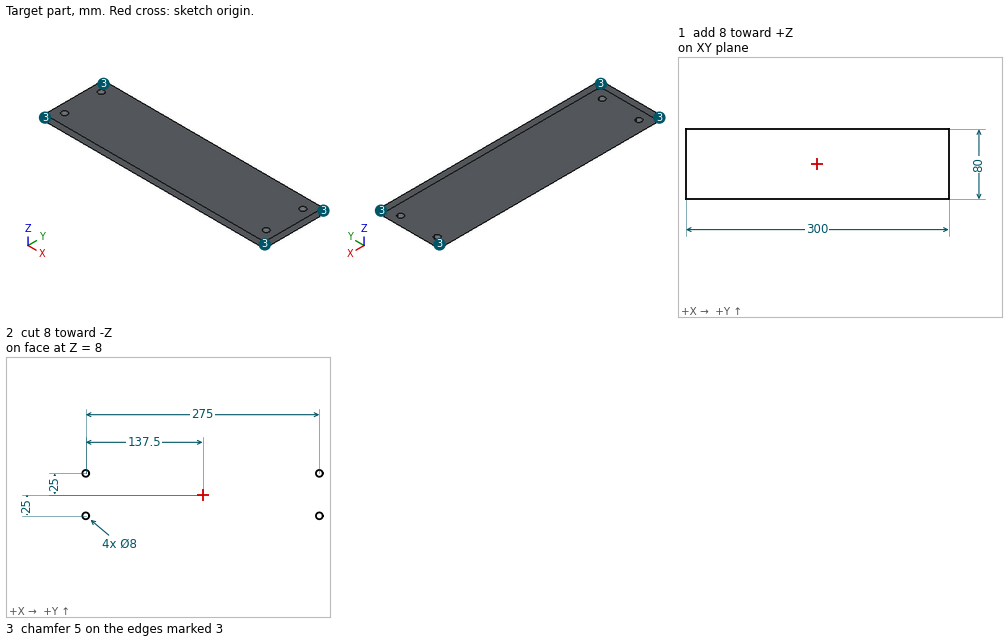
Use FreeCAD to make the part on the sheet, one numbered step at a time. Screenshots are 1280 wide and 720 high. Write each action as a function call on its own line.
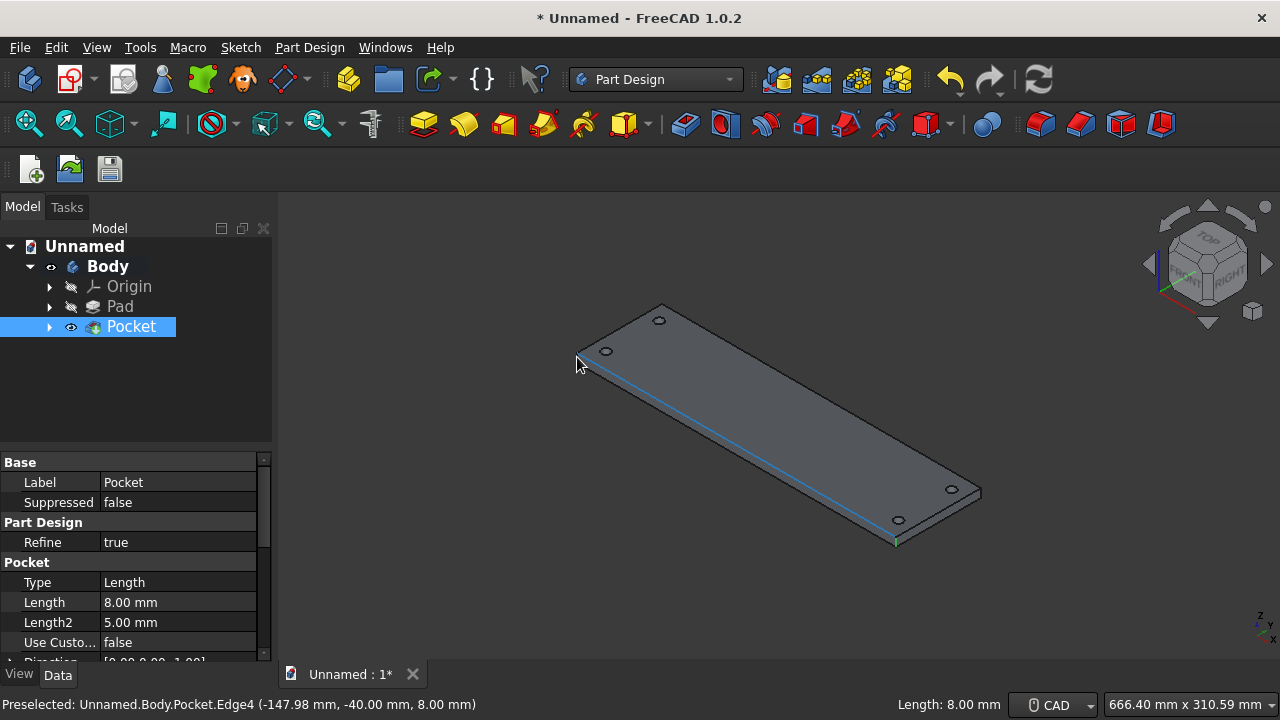
key(2)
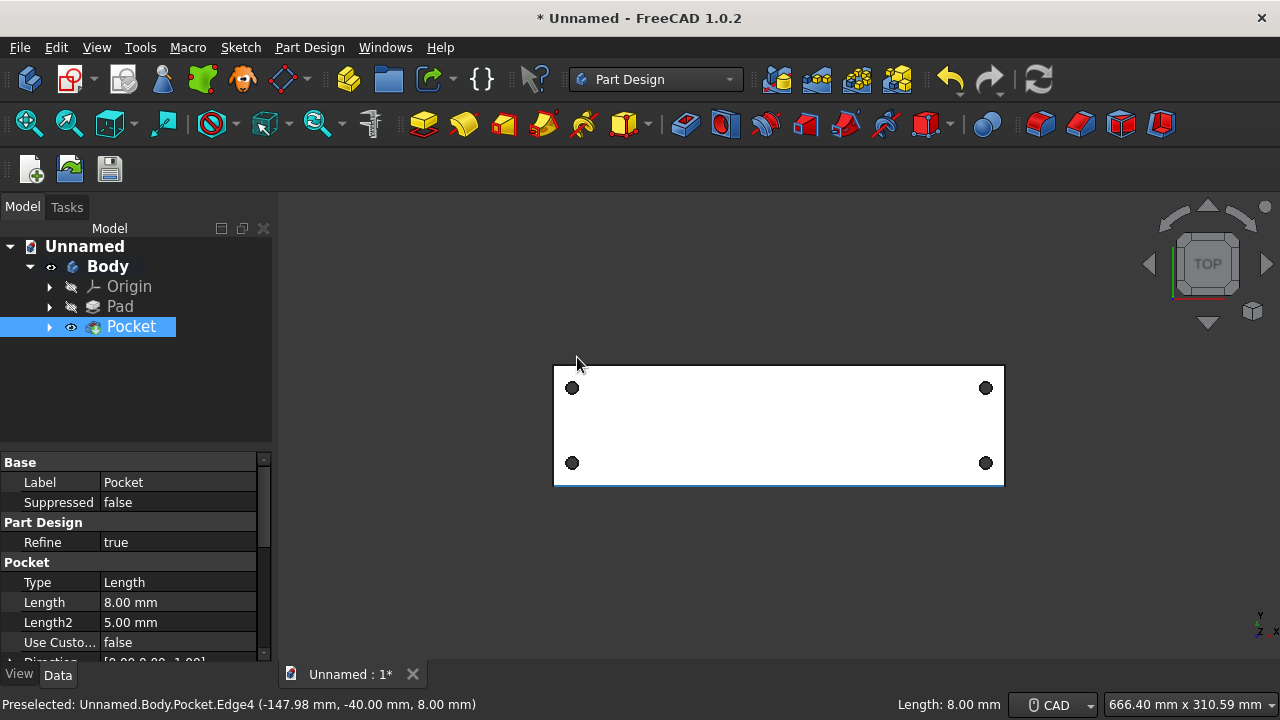
scroll(553, 485, up, 7)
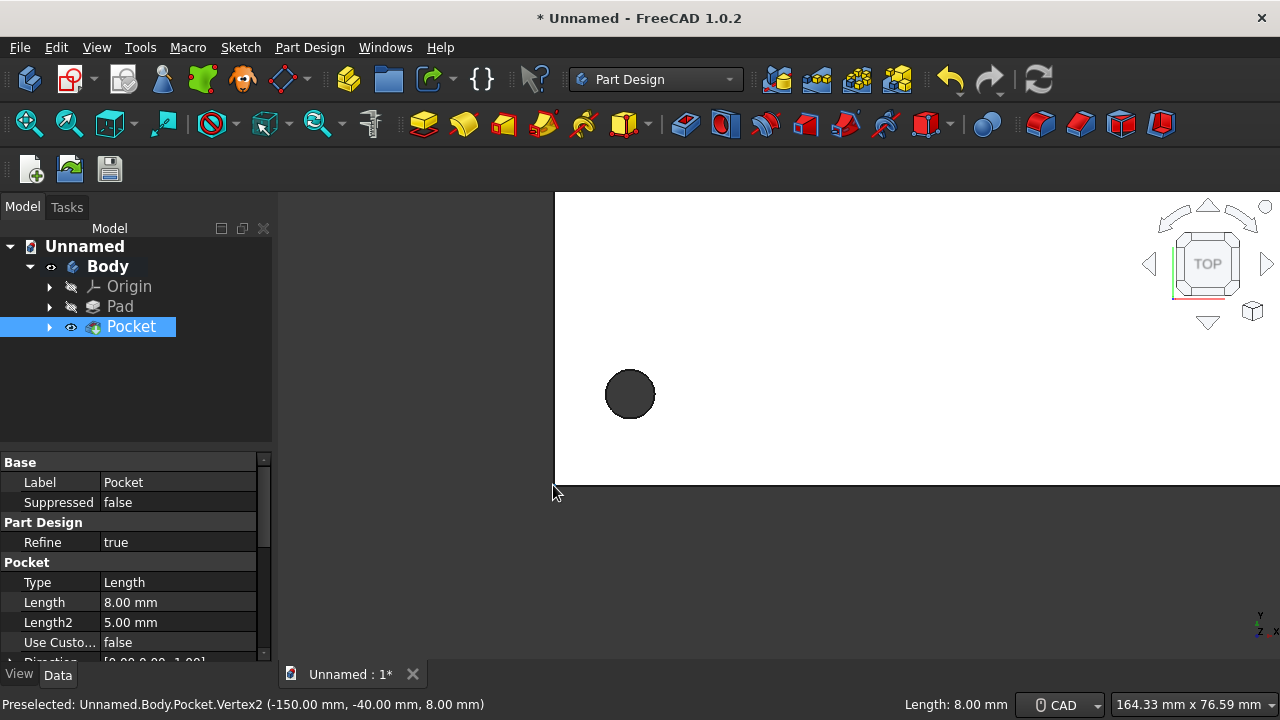
click(30, 124)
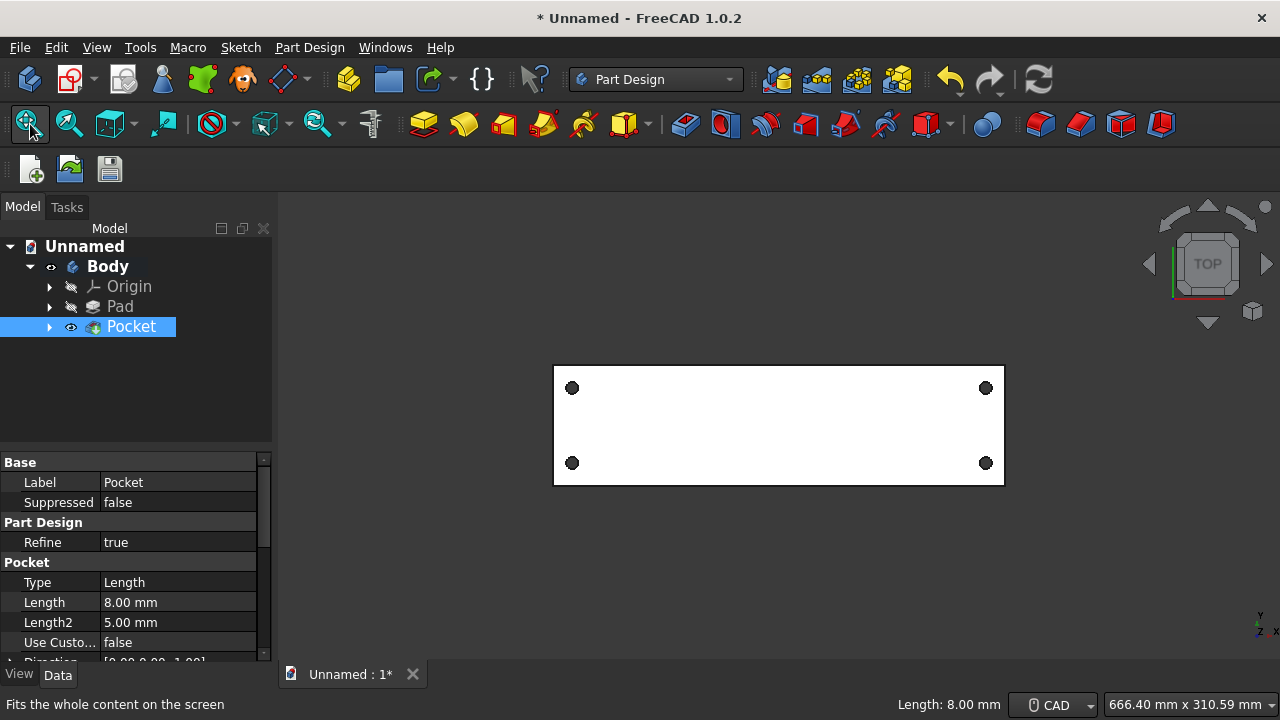
key(1)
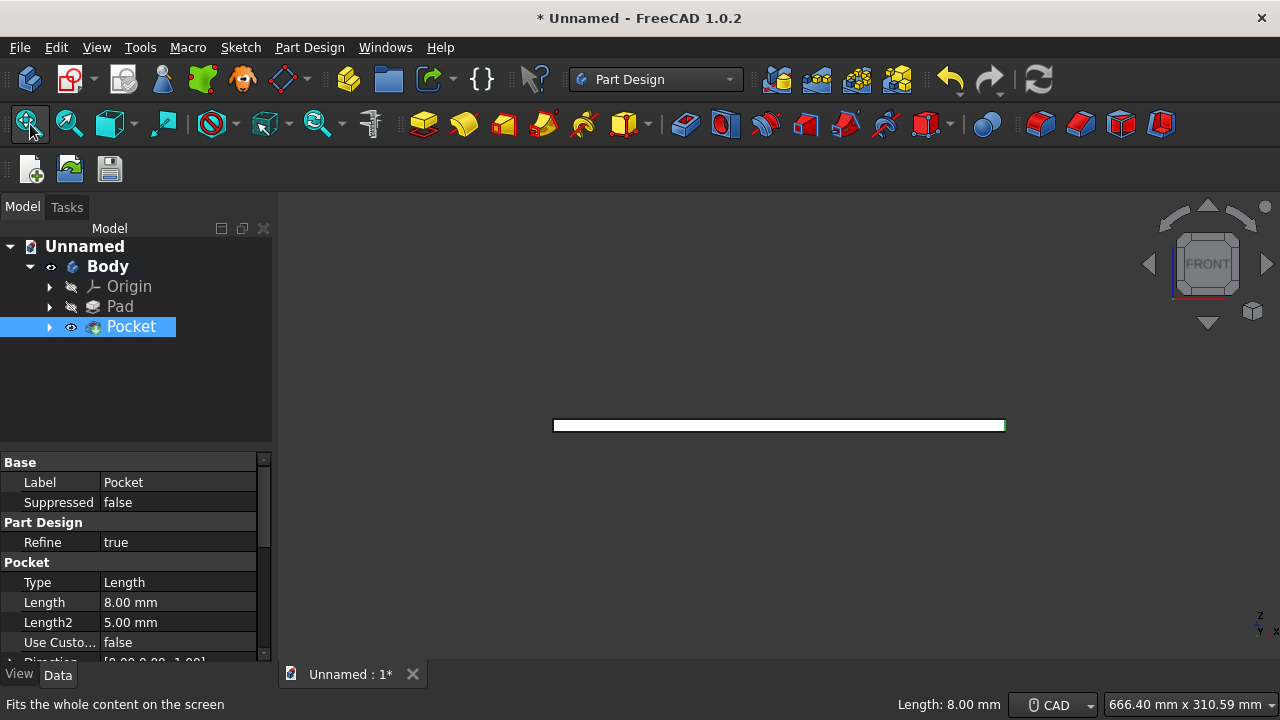
scroll(553, 425, up, 7)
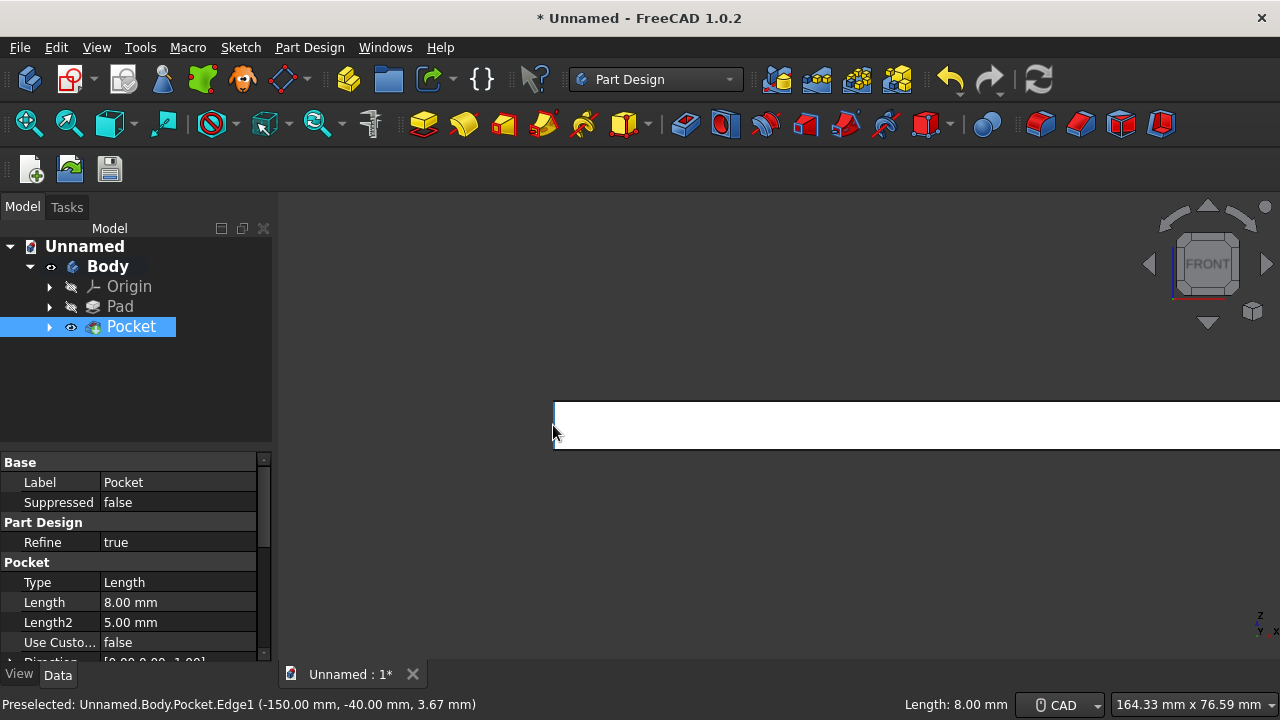
click(554, 425, ctrl)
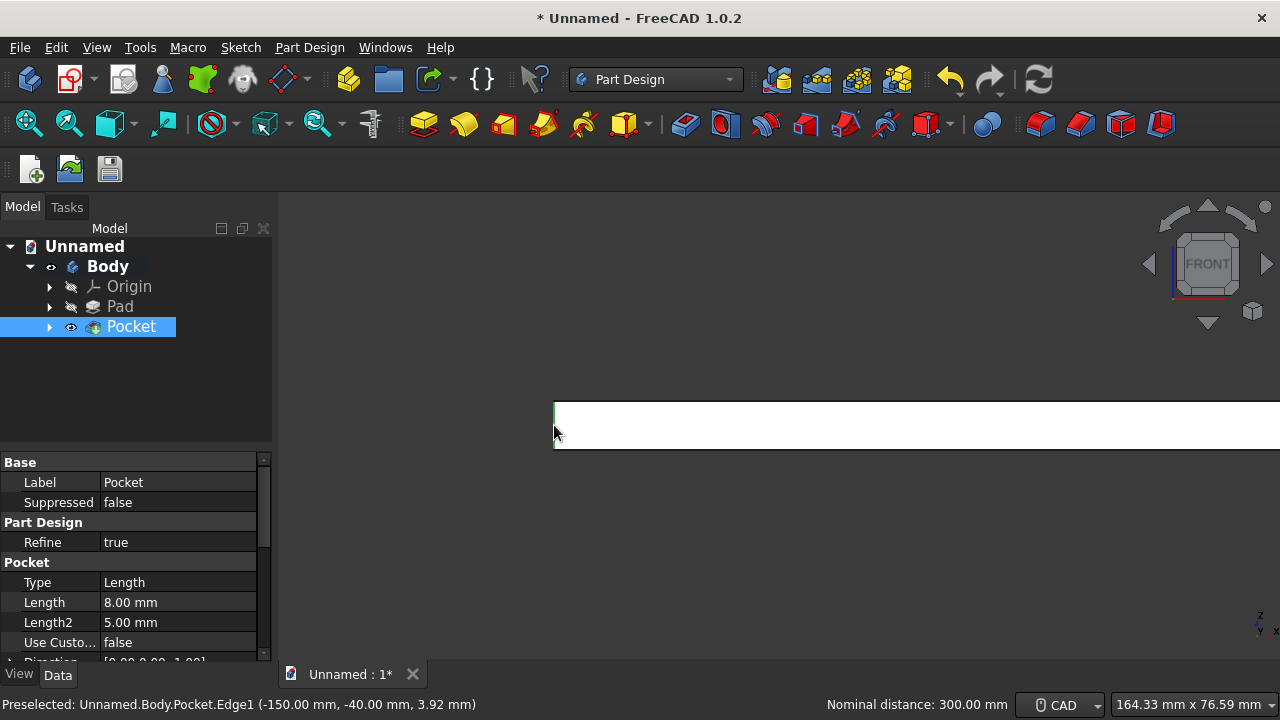
key(v)
key(f)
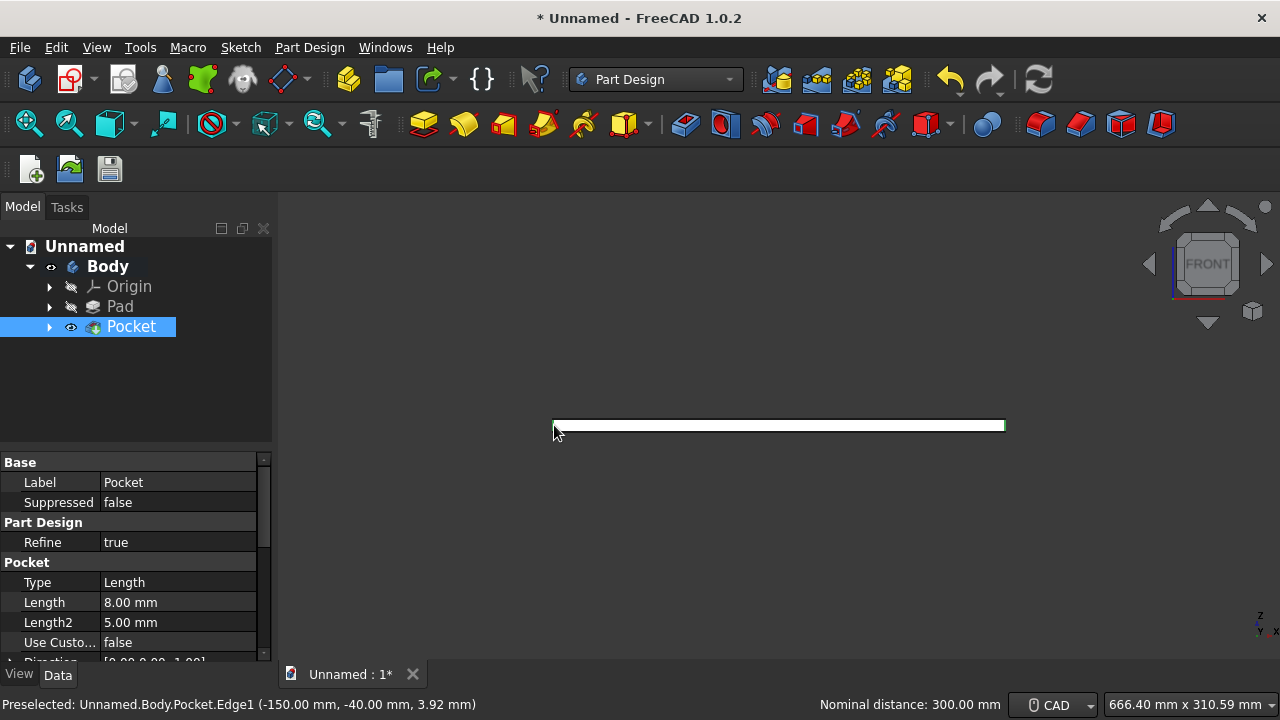
key(3)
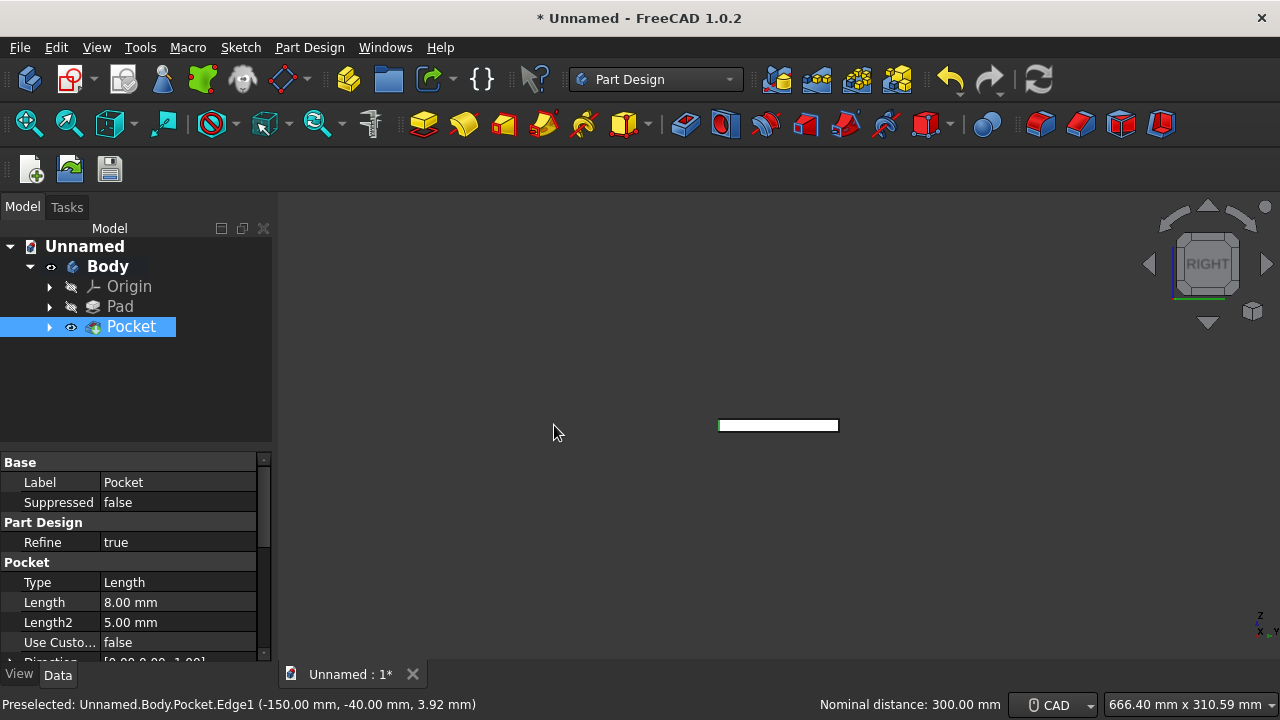
key(v)
key(f)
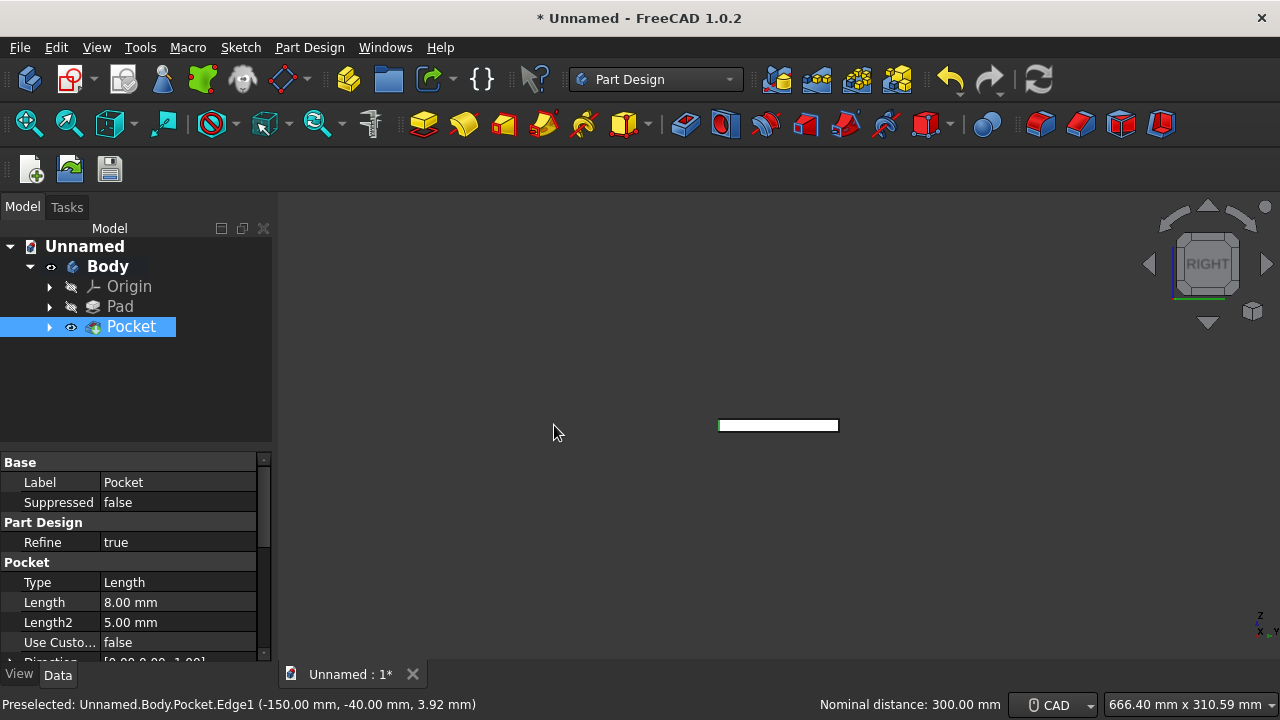
scroll(839, 424, up, 7)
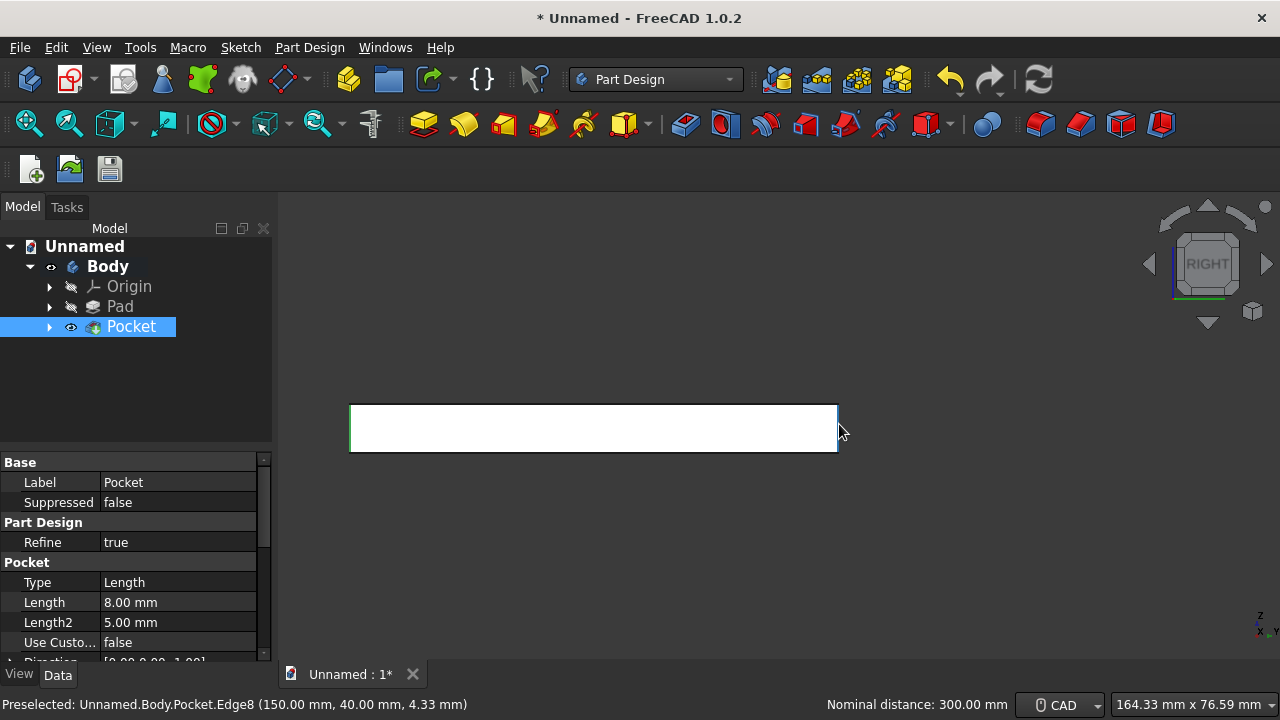
click(838, 428, ctrl)